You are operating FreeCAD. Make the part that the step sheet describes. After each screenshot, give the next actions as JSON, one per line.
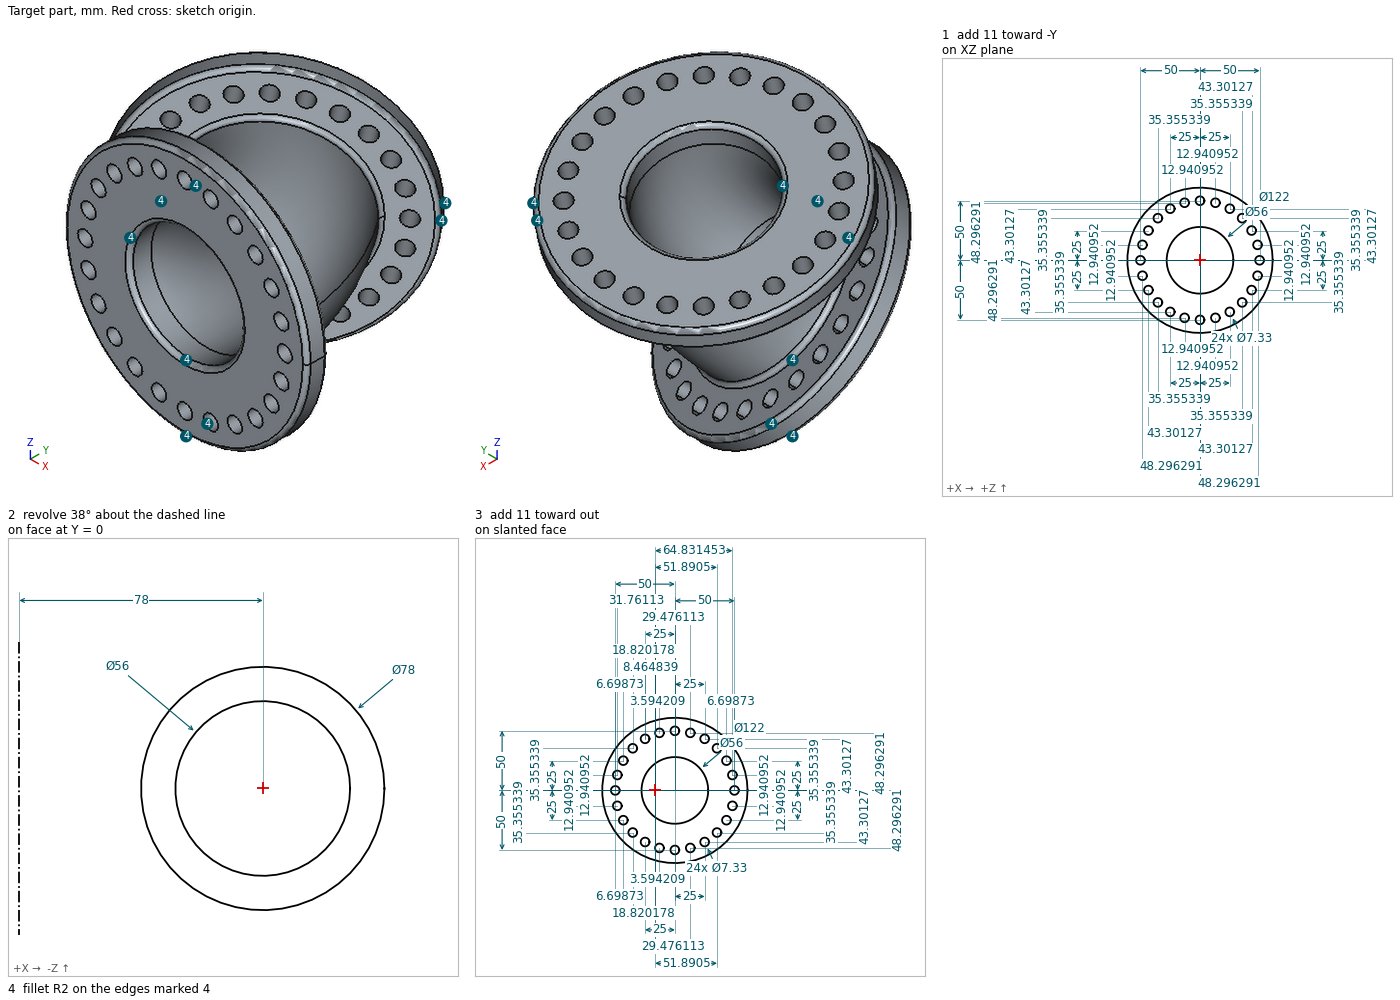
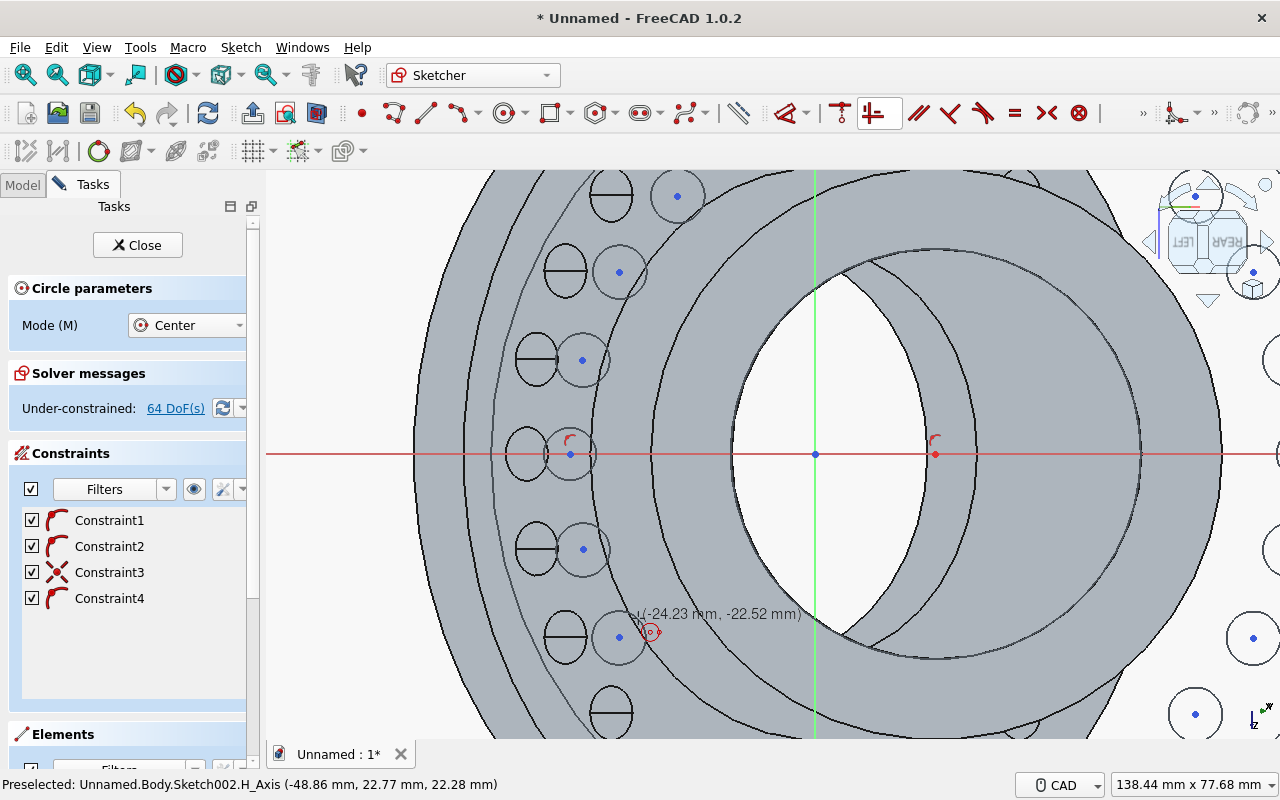
{"action": "scroll", "coordinate": [569, 455], "scroll_direction": "down", "scroll_amount": 5}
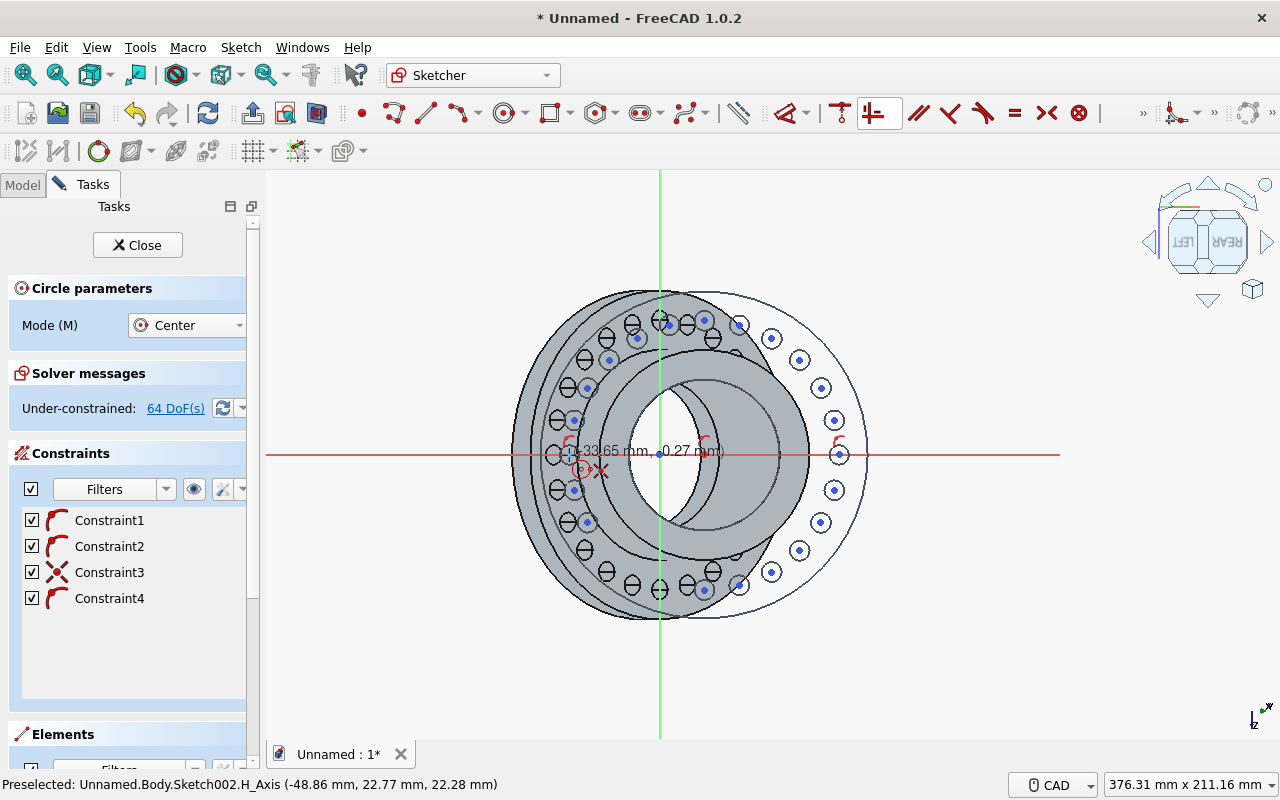
{"action": "scroll", "coordinate": [670, 585], "scroll_direction": "up", "scroll_amount": 5}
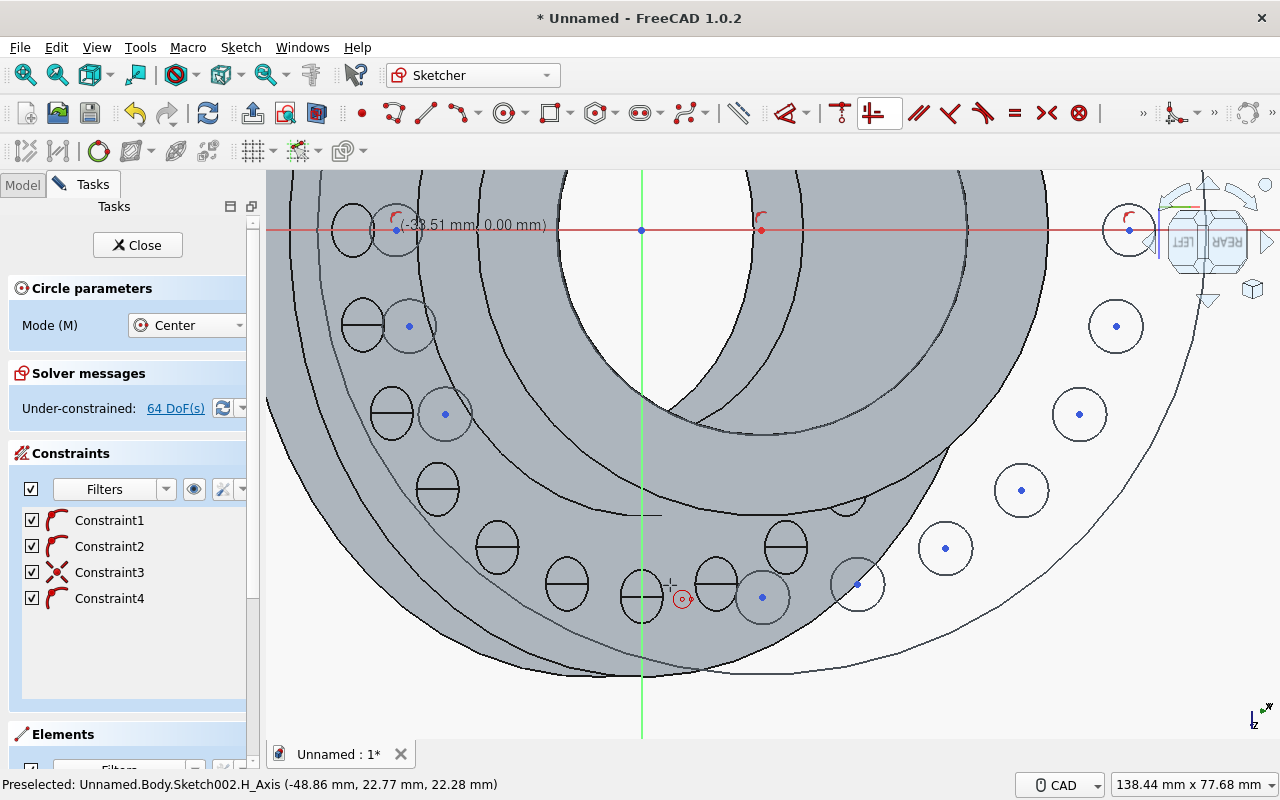
{"action": "left_click", "coordinate": [668, 584]}
{"action": "left_click", "coordinate": [687, 565]}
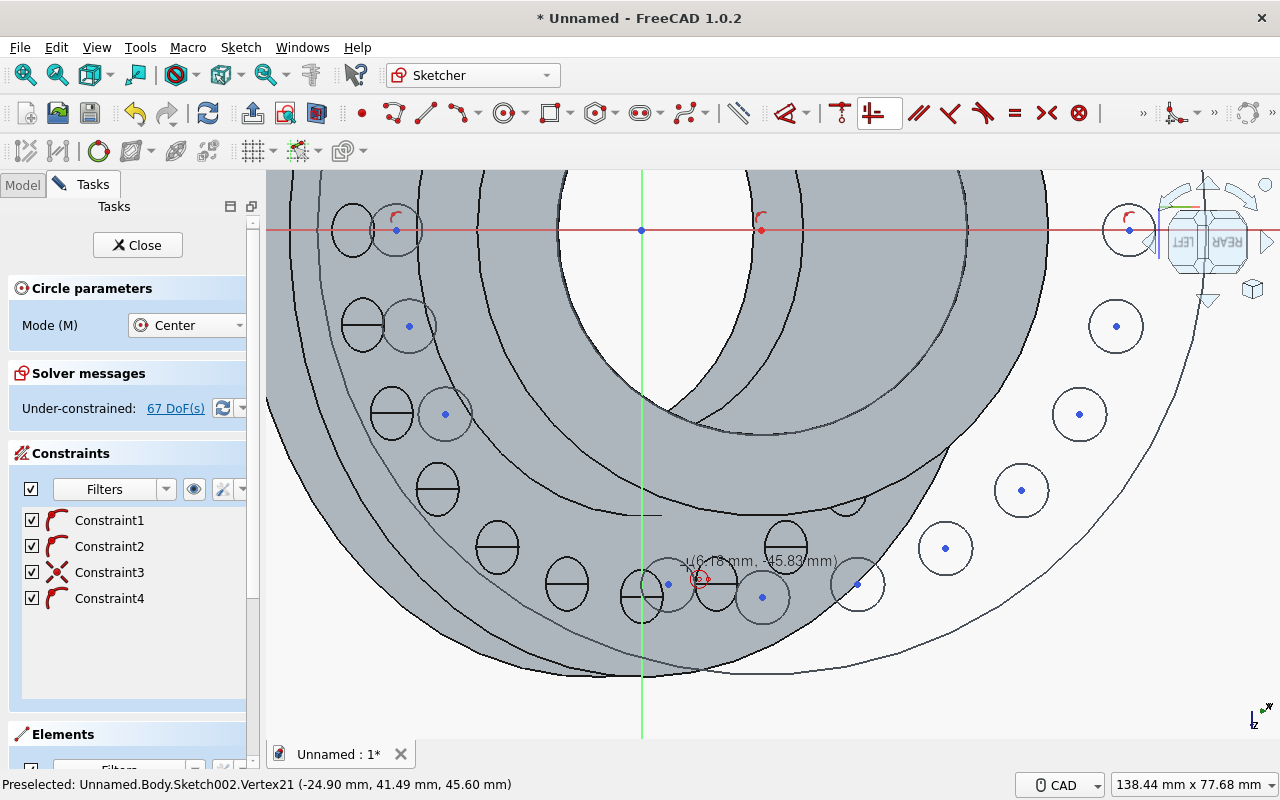
{"action": "left_click", "coordinate": [580, 547]}
{"action": "left_click", "coordinate": [599, 528]}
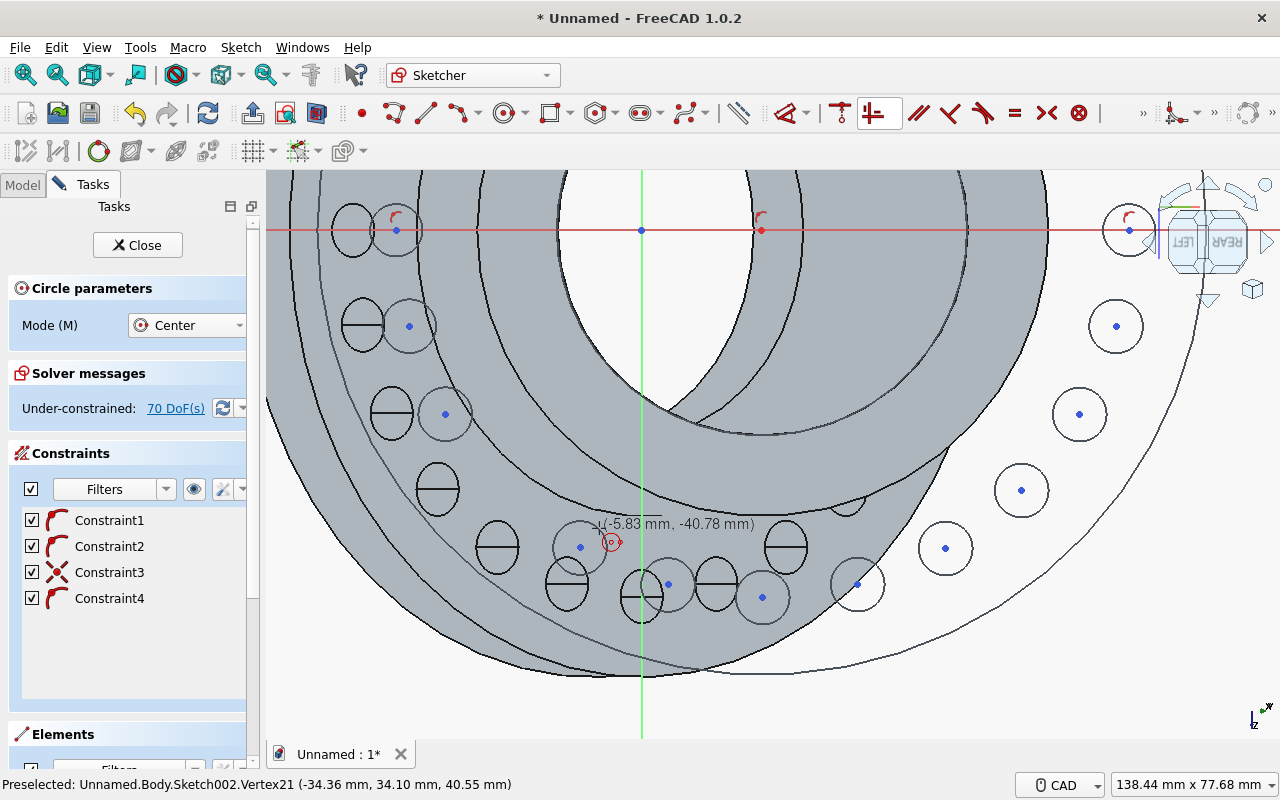
{"action": "left_click", "coordinate": [504, 489]}
{"action": "left_click", "coordinate": [523, 470]}
{"action": "key", "text": "Escape"}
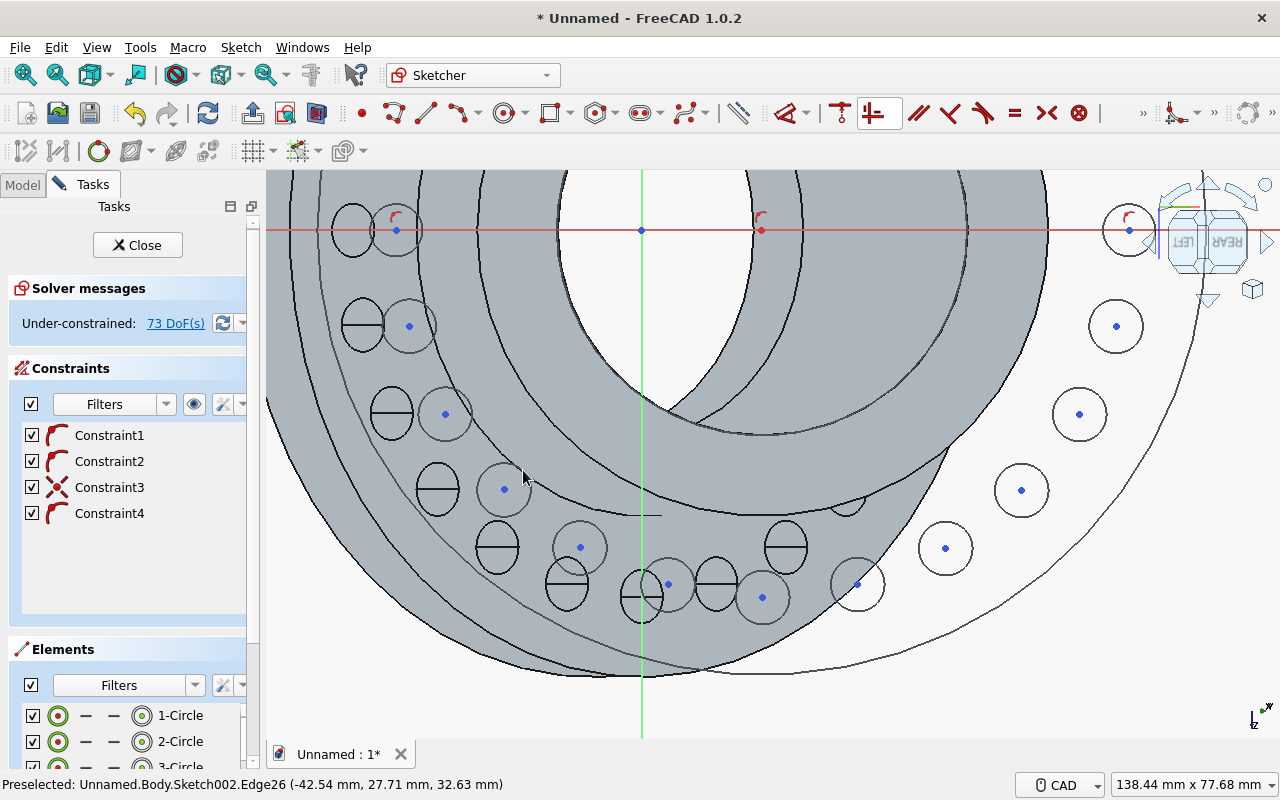
{"action": "scroll", "coordinate": [671, 585], "scroll_direction": "down", "scroll_amount": 5}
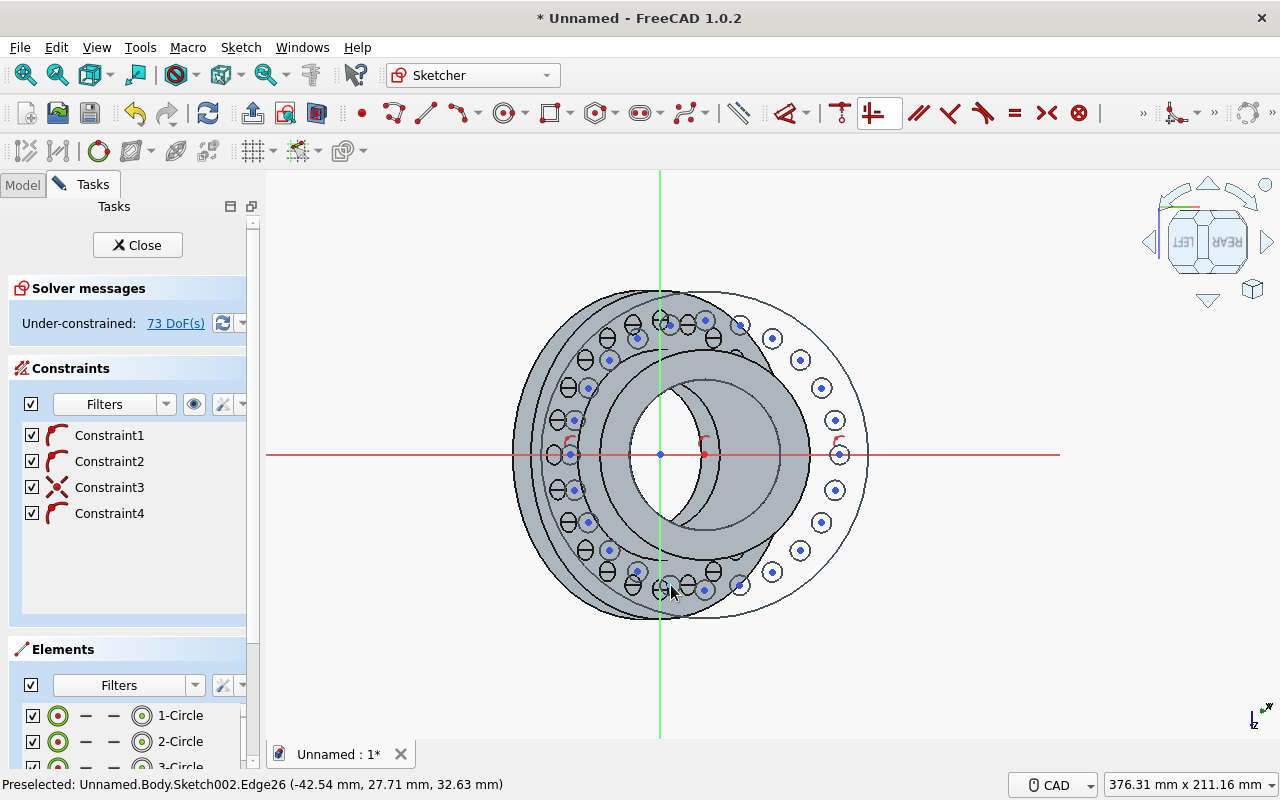
{"action": "scroll", "coordinate": [807, 353], "scroll_direction": "up", "scroll_amount": 2}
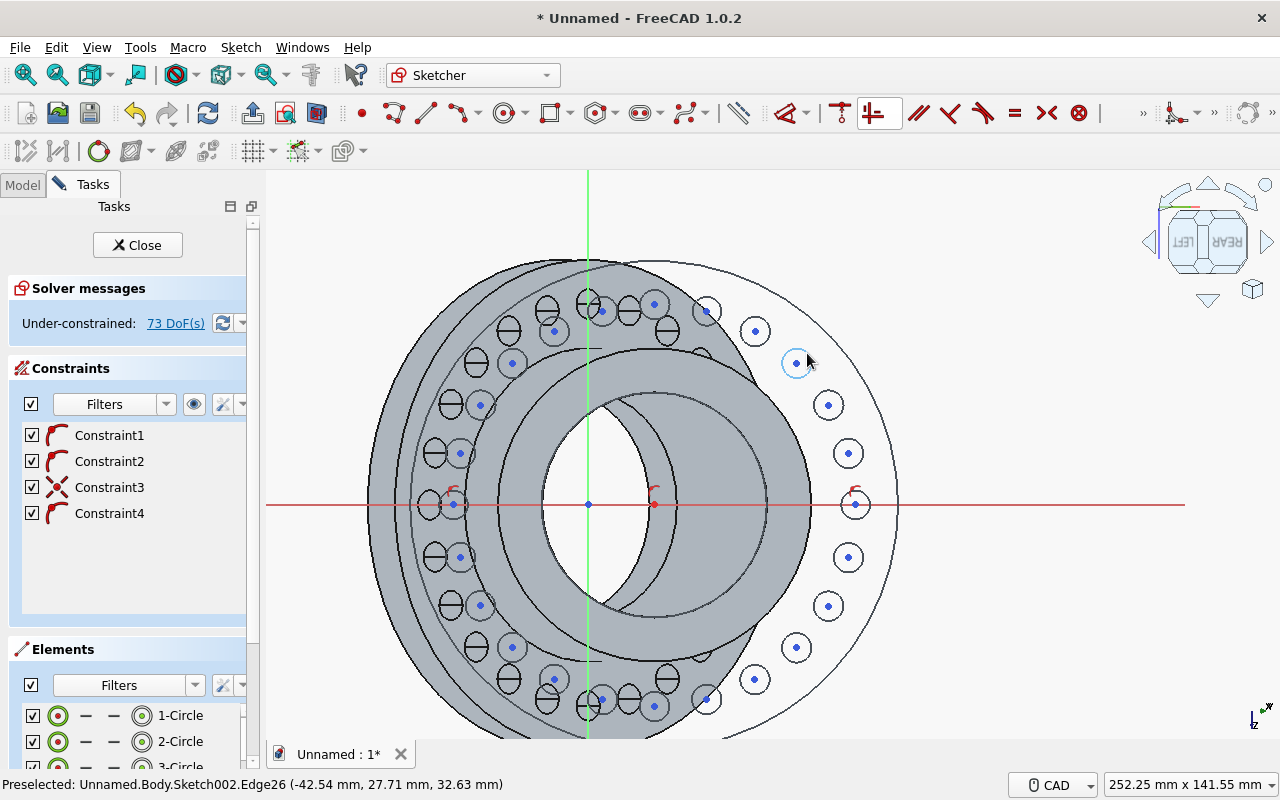
{"action": "left_click", "coordinate": [807, 353]}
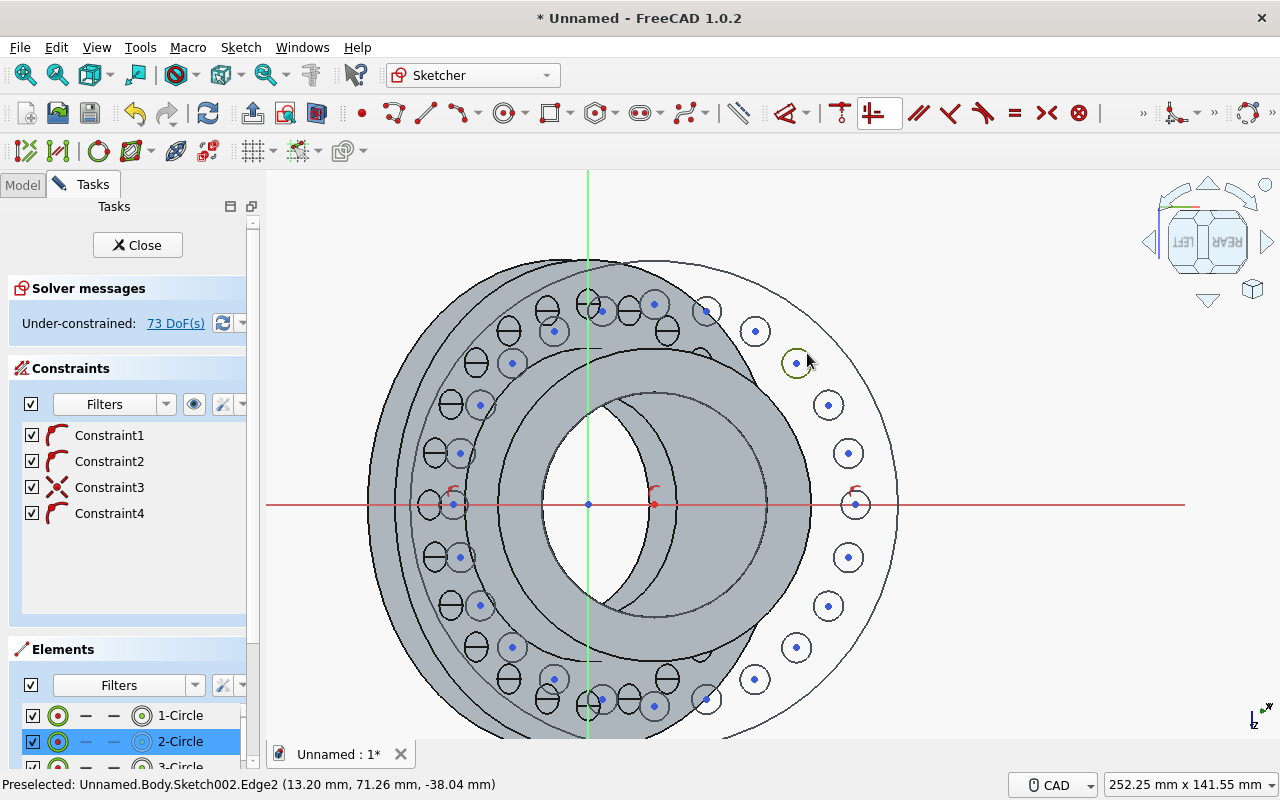
{"action": "left_click", "coordinate": [766, 321]}